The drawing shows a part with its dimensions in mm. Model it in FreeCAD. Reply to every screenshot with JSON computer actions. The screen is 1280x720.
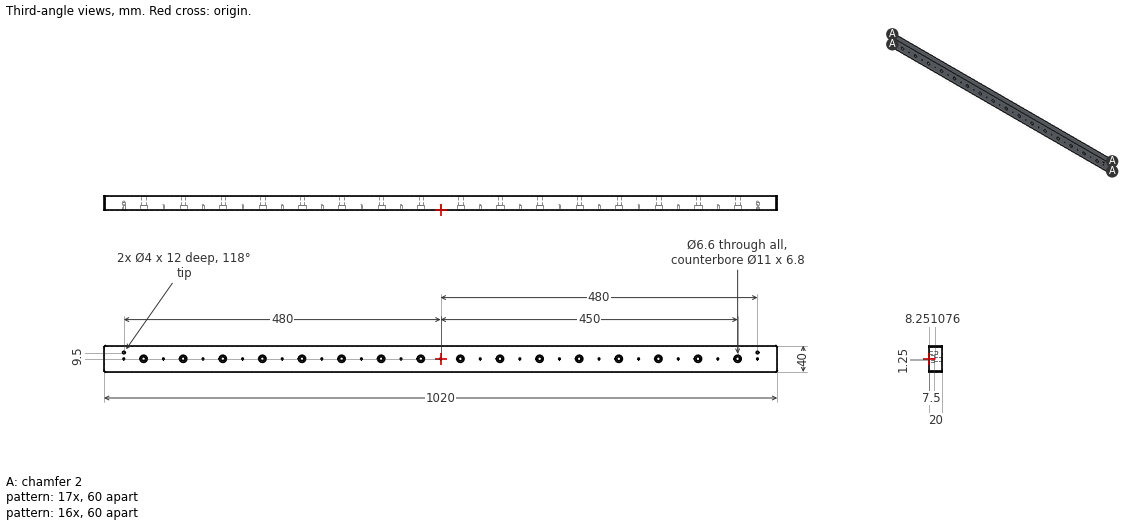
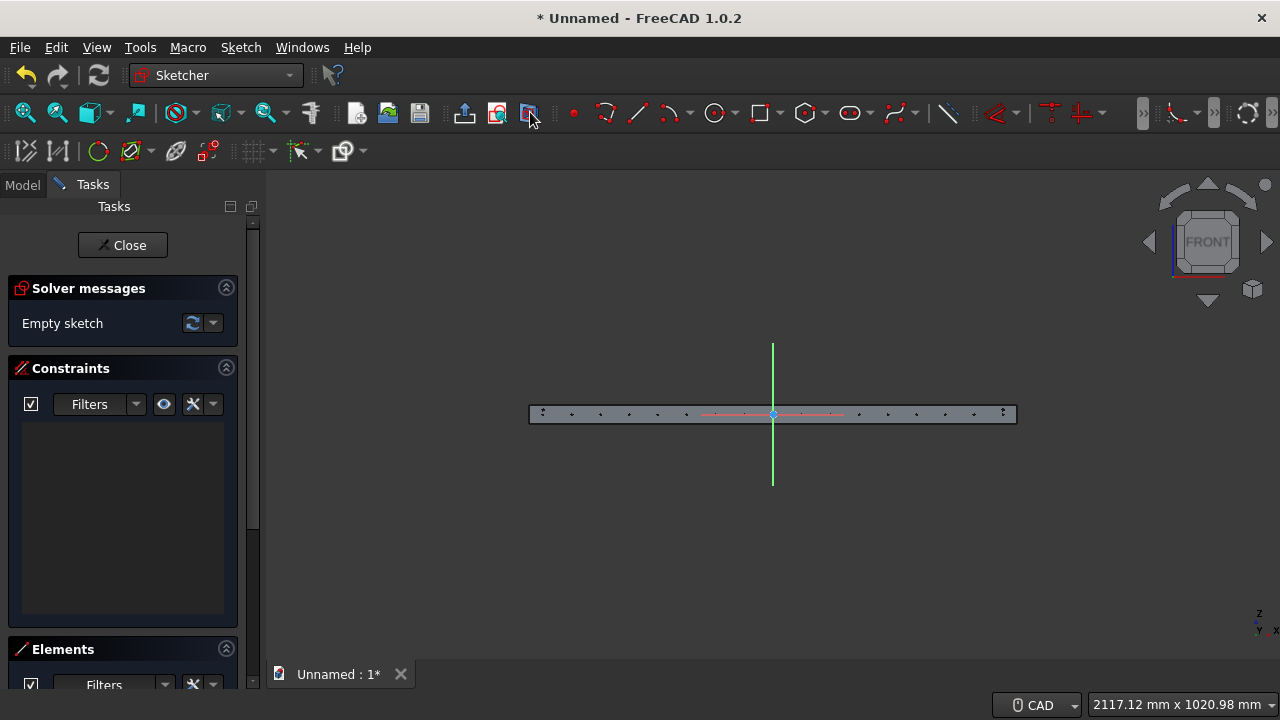
{"action": "scroll", "coordinate": [1003, 414], "scroll_direction": "up", "scroll_amount": 15}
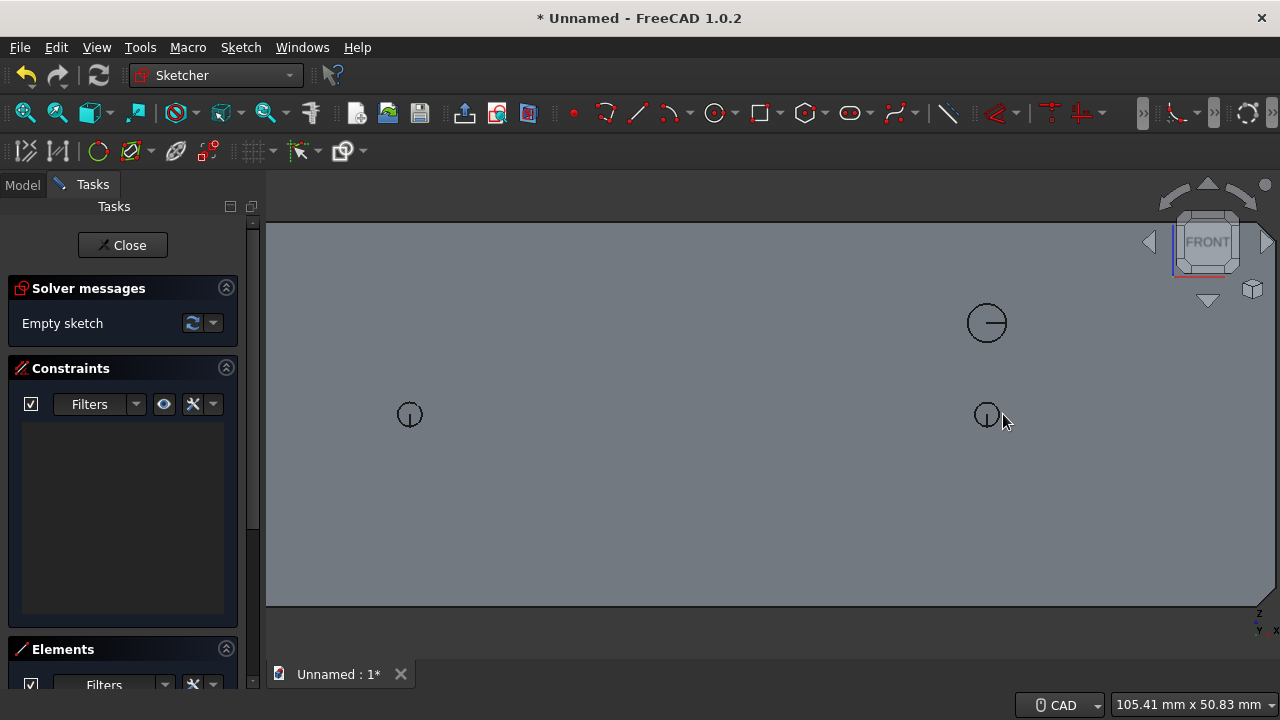
{"action": "scroll", "coordinate": [697, 414], "scroll_direction": "up", "scroll_amount": 8}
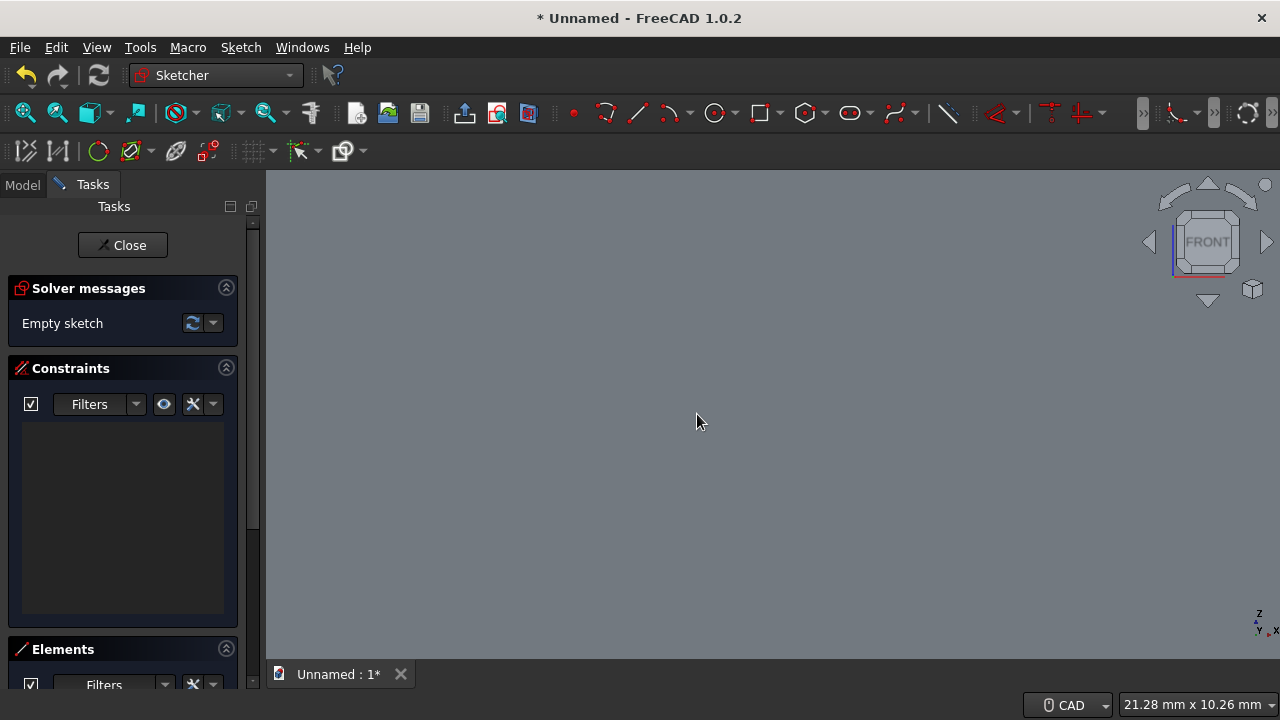
{"action": "key", "text": "g c"}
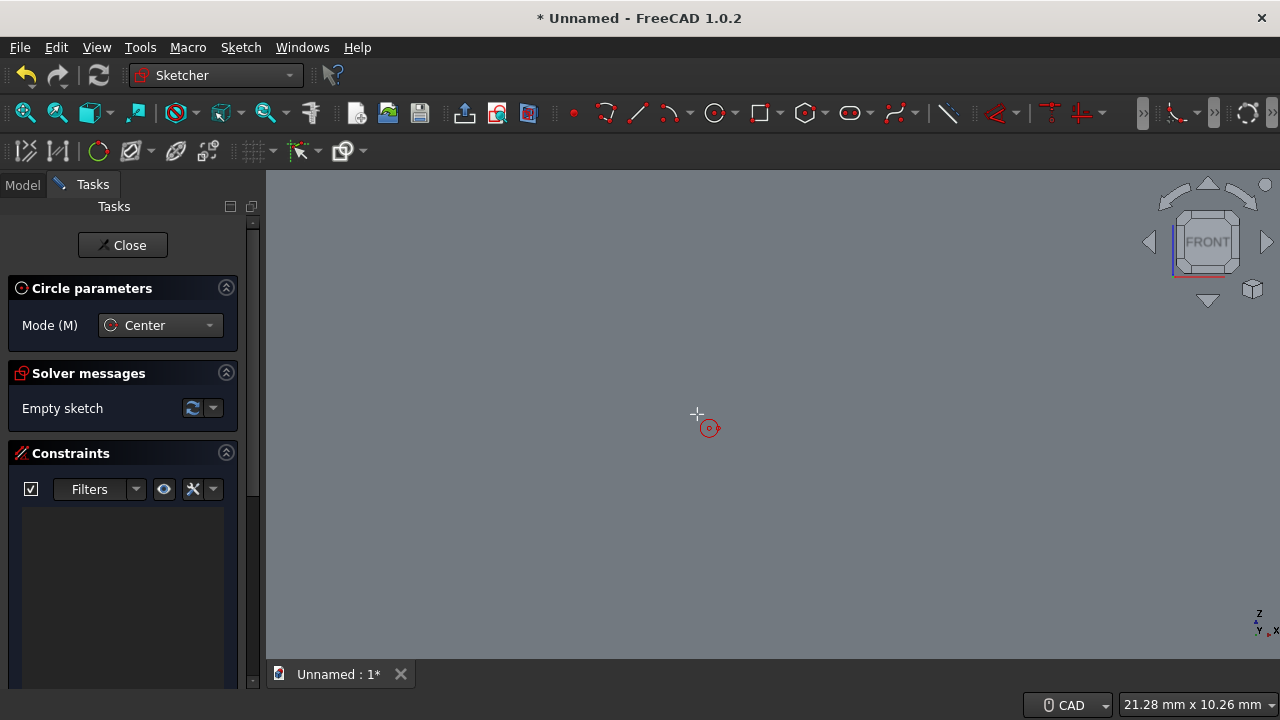
{"action": "left_click", "coordinate": [702, 414]}
{"action": "mouse_move", "coordinate": [814, 303]}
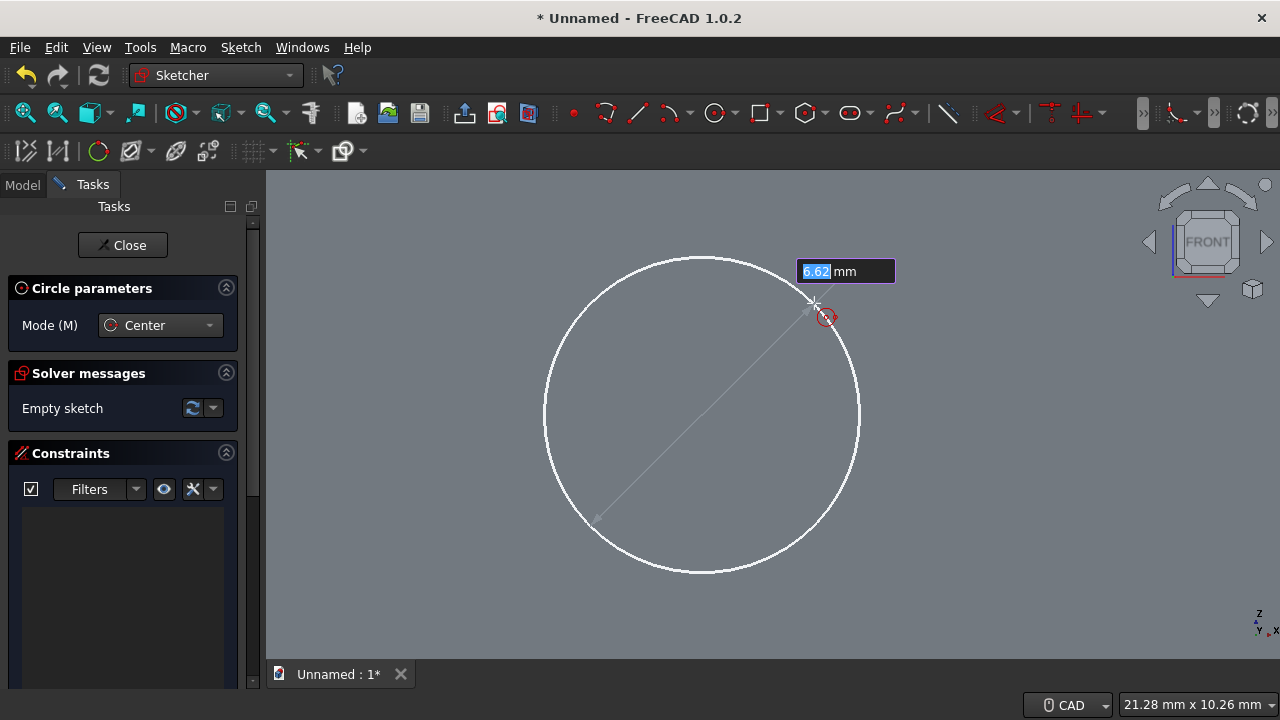
{"action": "type", "text": "6.6"}
{"action": "key", "text": "Return"}
{"action": "key", "text": "Escape"}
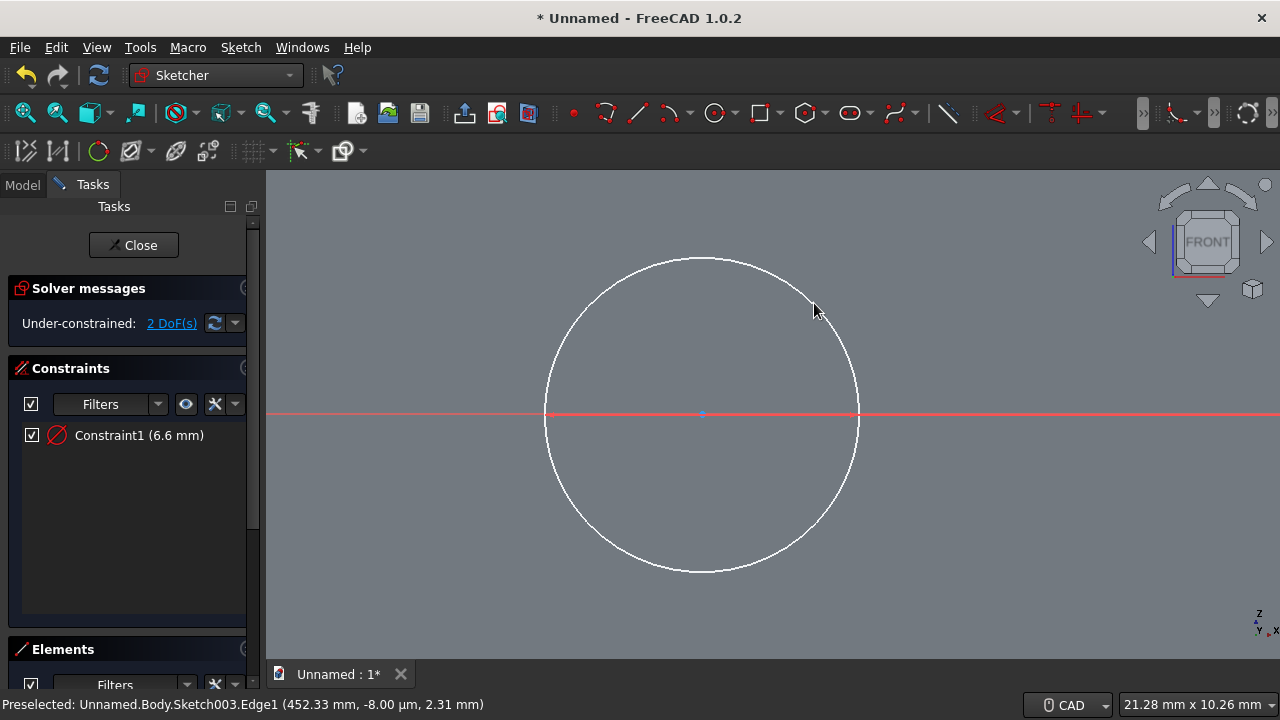
{"action": "left_click", "coordinate": [702, 415]}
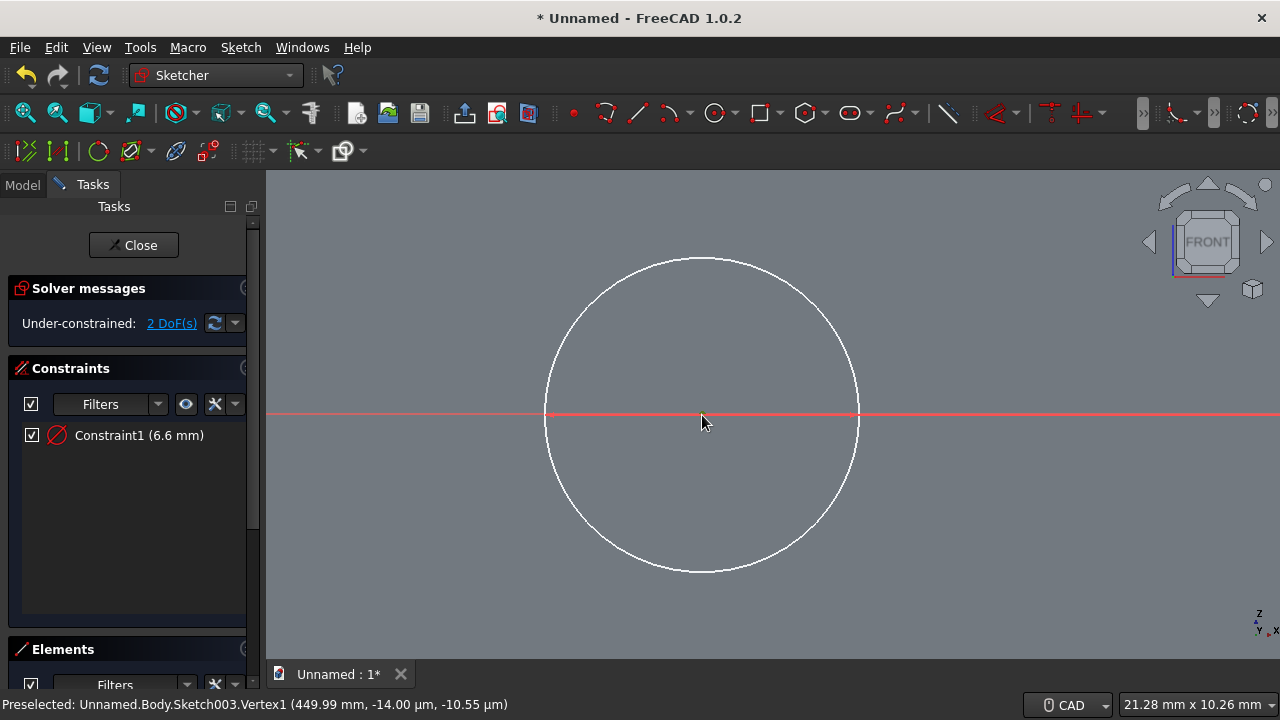
{"action": "left_click", "coordinate": [353, 414]}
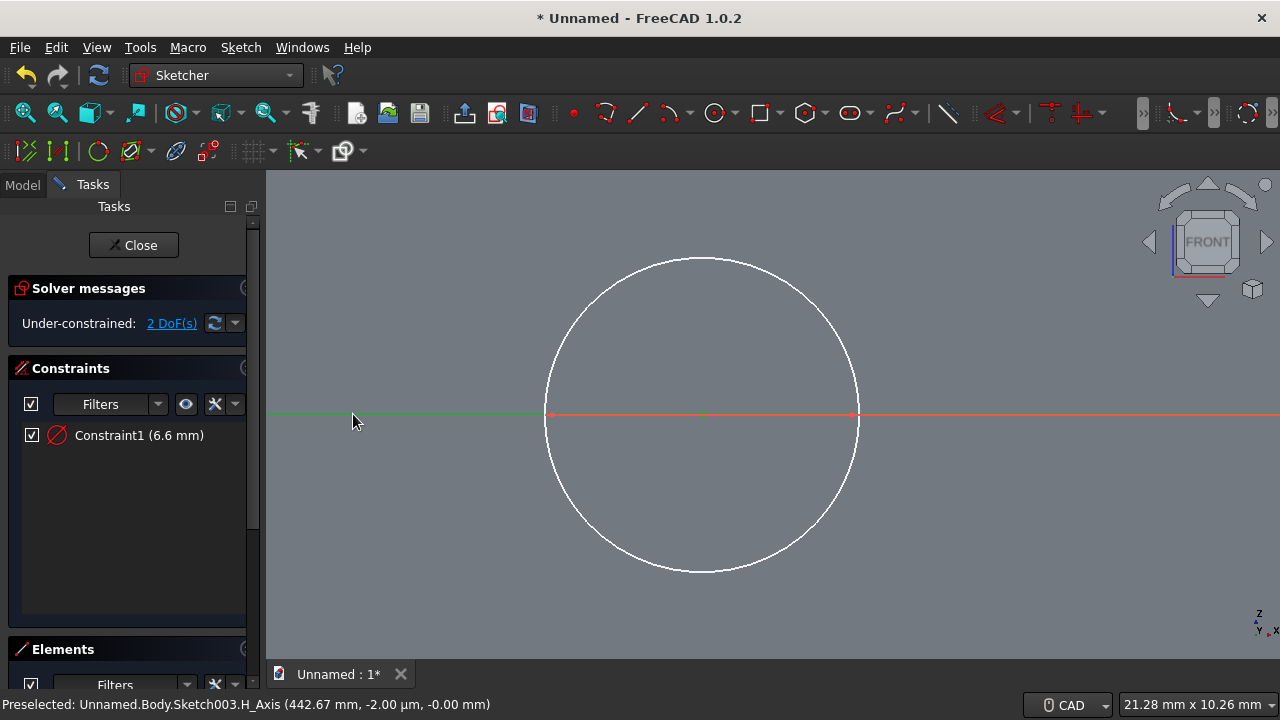
{"action": "key", "text": "c"}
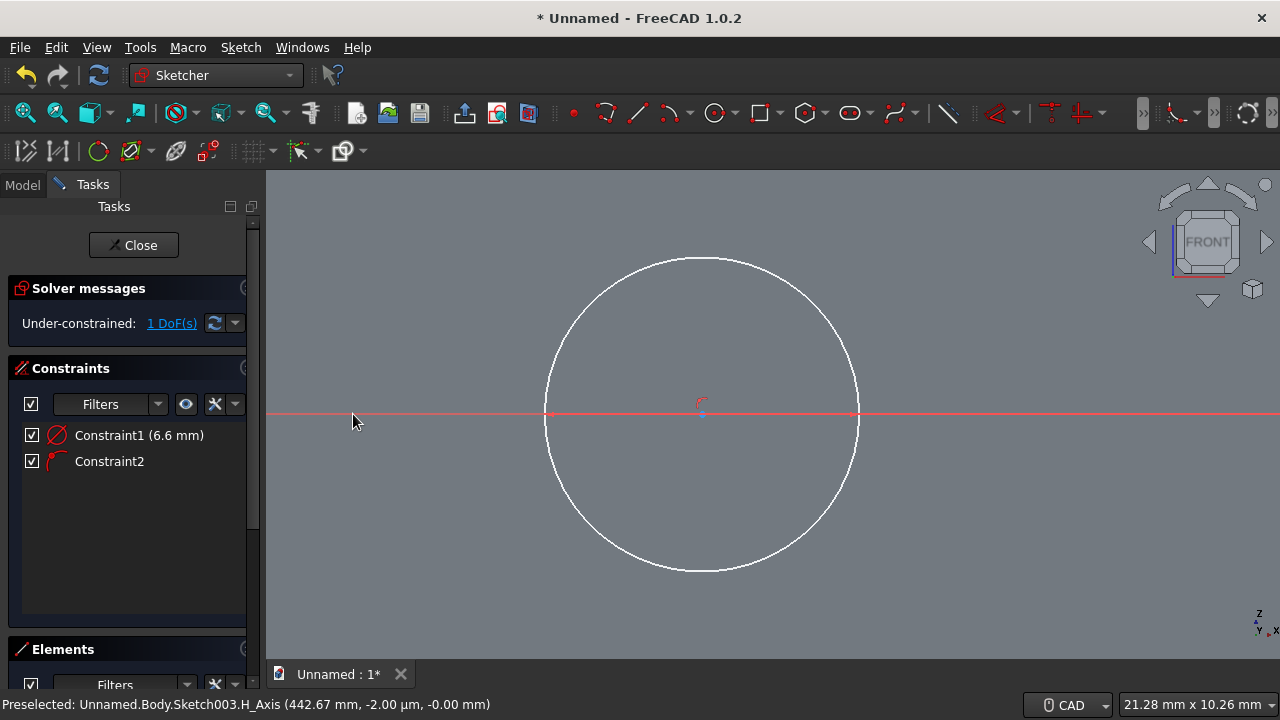
{"action": "key", "text": "d"}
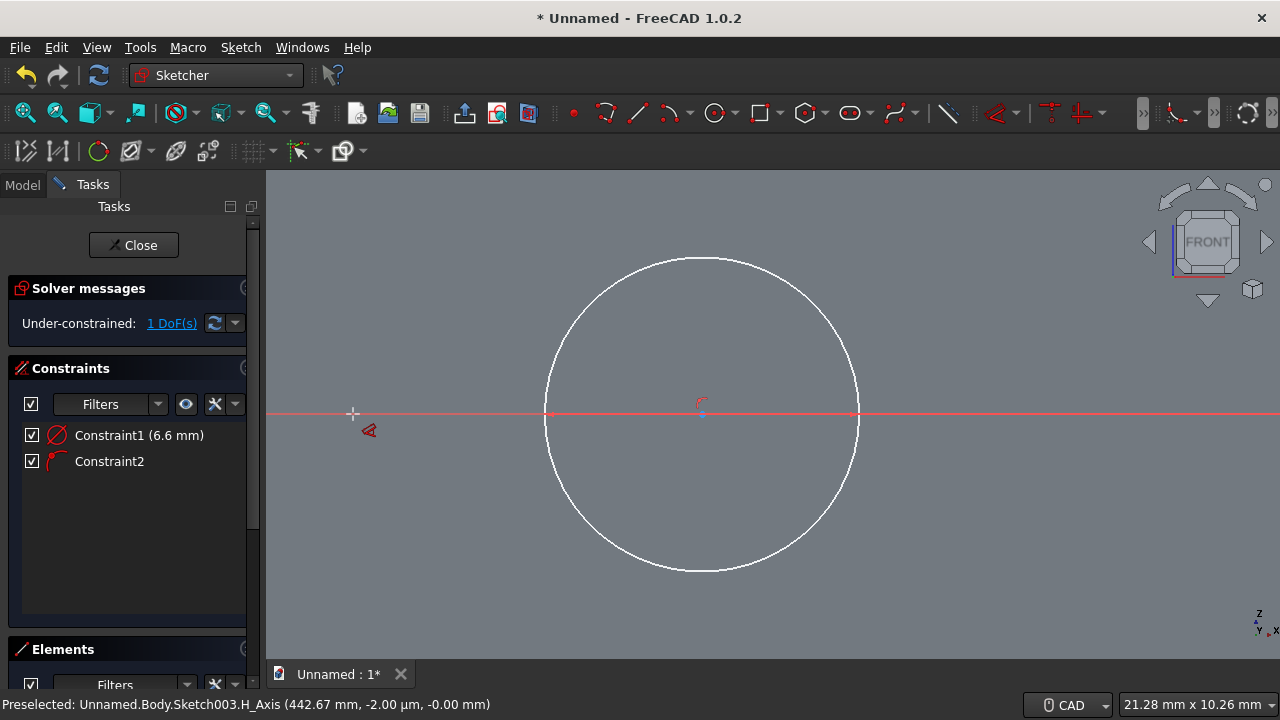
{"action": "left_click", "coordinate": [702, 414]}
{"action": "left_click", "coordinate": [498, 448]}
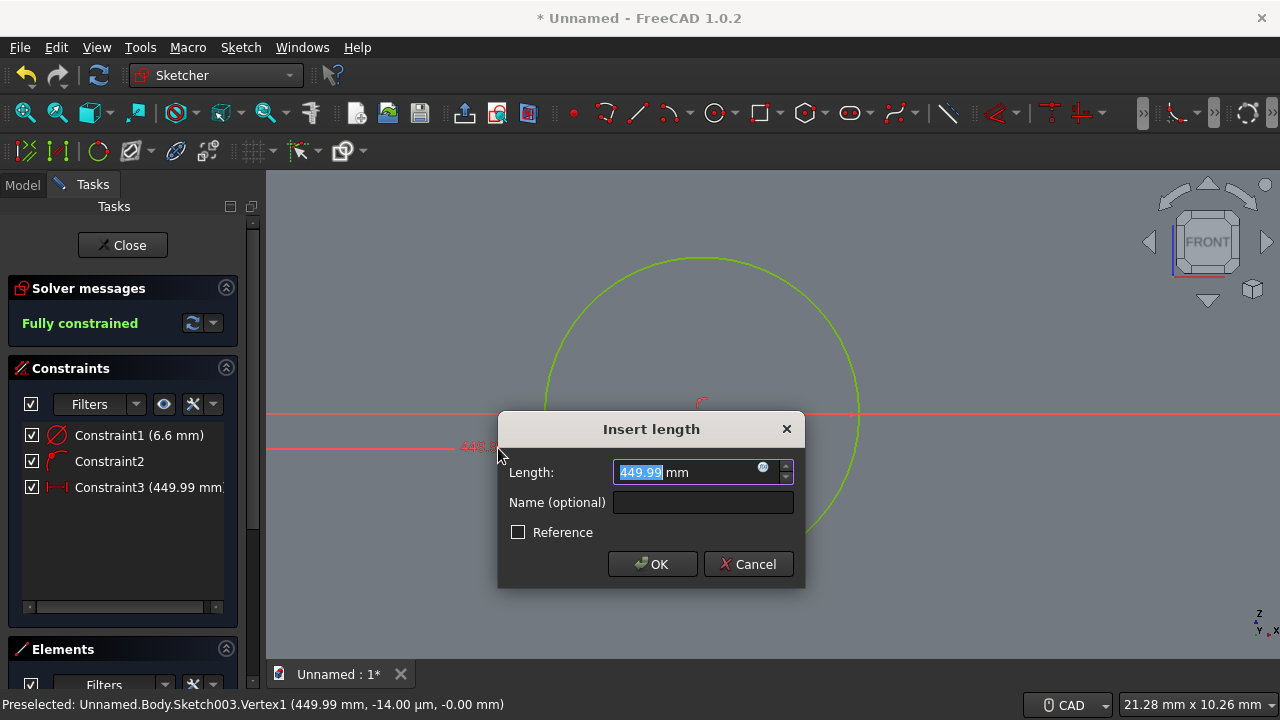
{"action": "type", "text": "450"}
{"action": "key", "text": "Return"}
{"action": "key", "text": "Escape"}